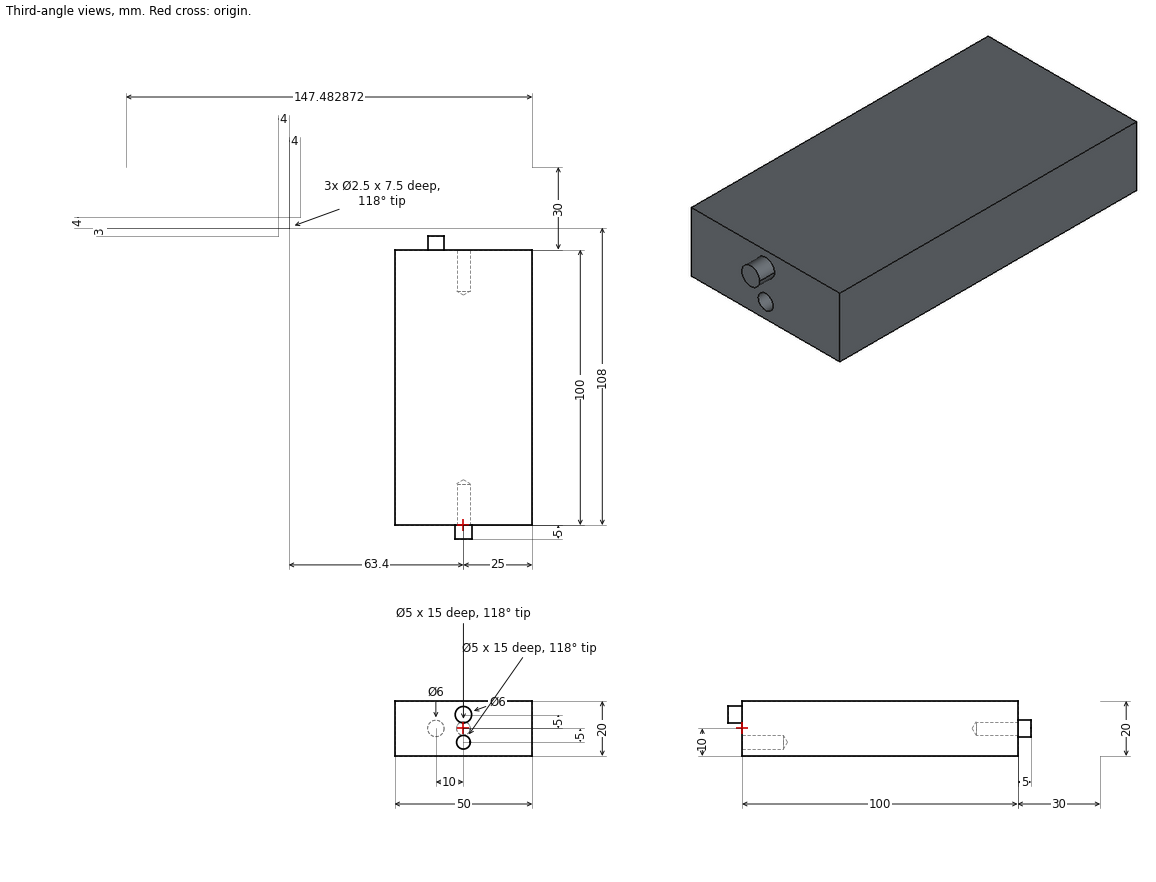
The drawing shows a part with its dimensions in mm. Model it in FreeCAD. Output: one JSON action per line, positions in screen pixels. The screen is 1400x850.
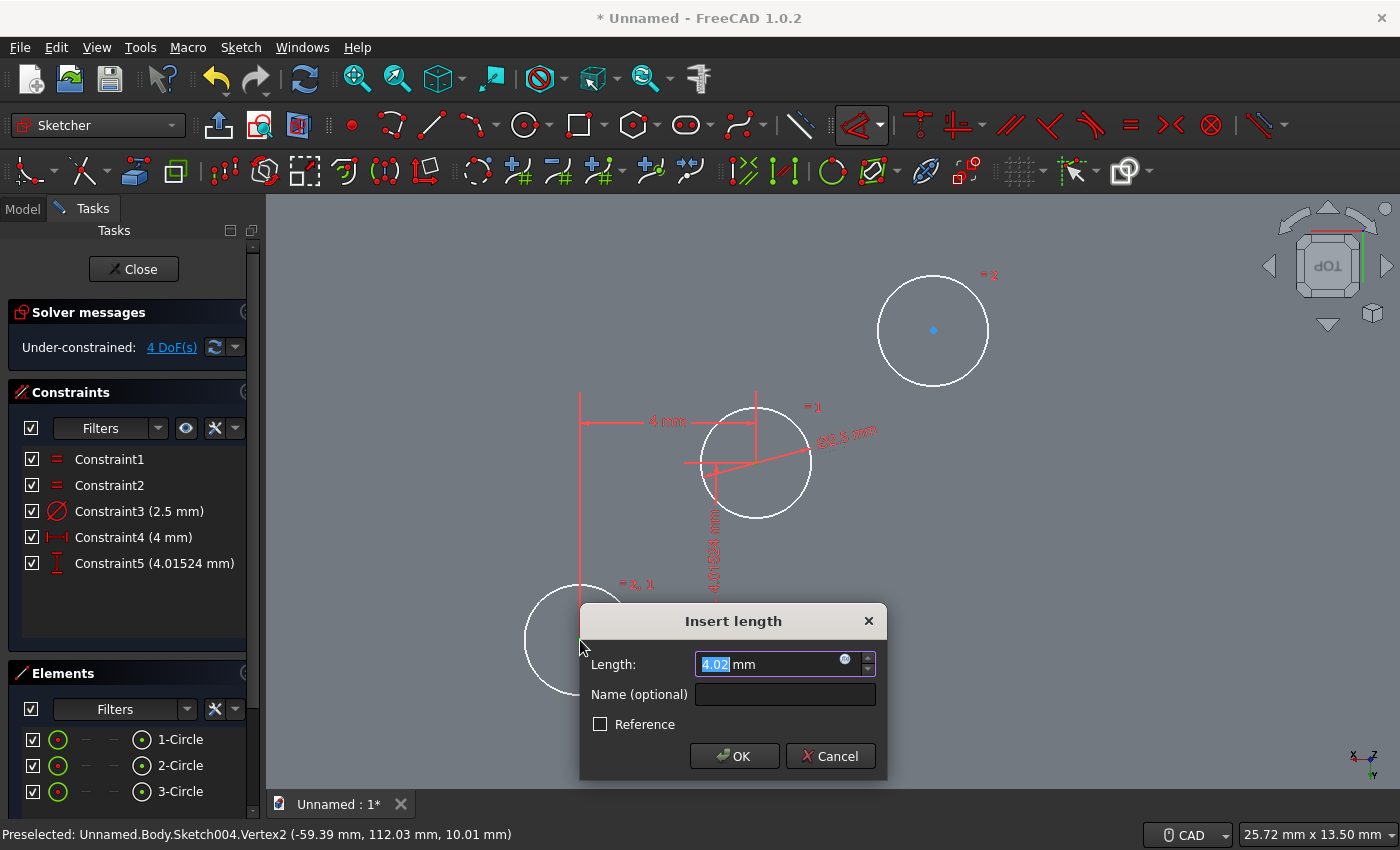
{"action": "type", "text": "4"}
{"action": "key", "text": "Return"}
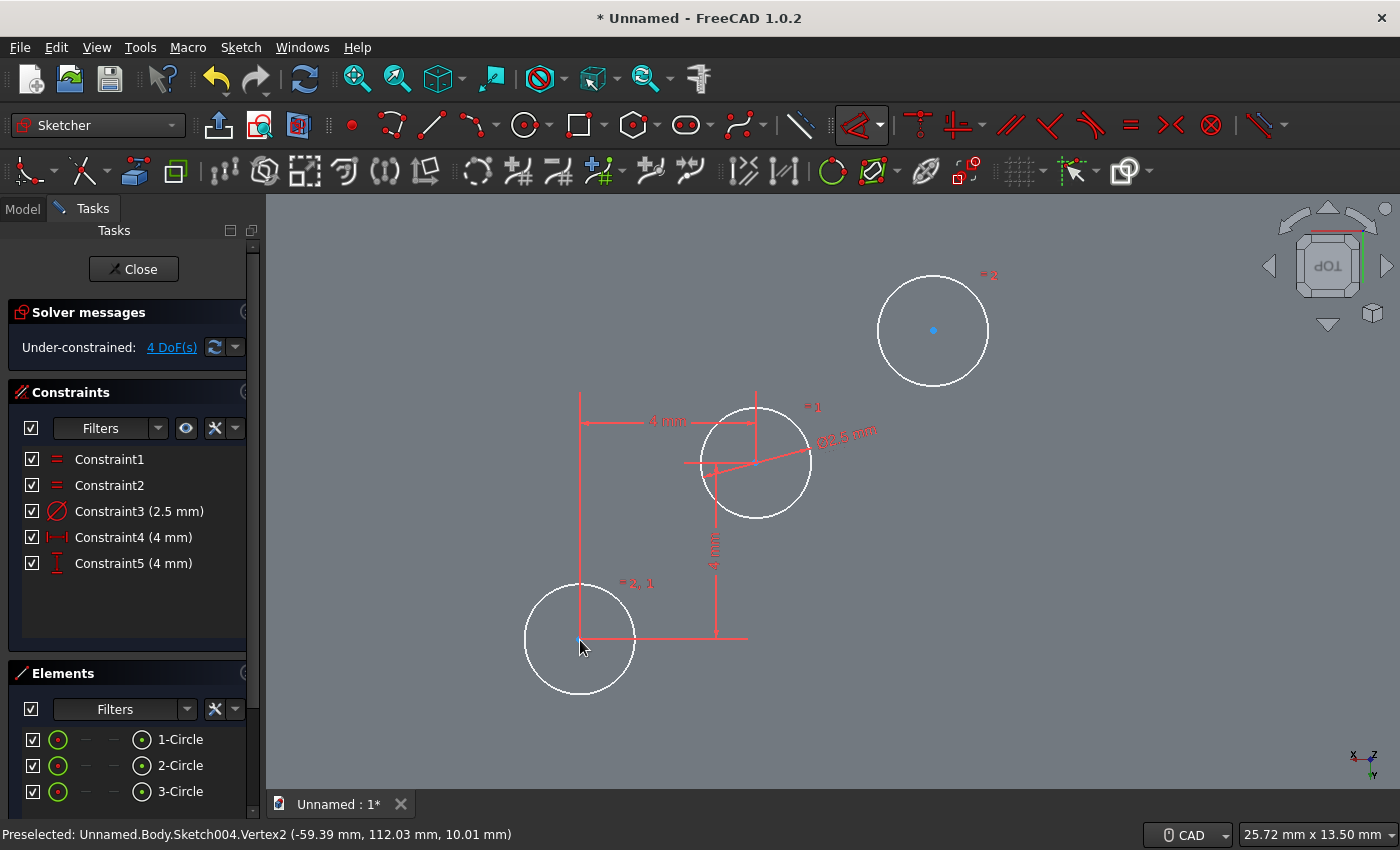
{"action": "left_click", "coordinate": [756, 463]}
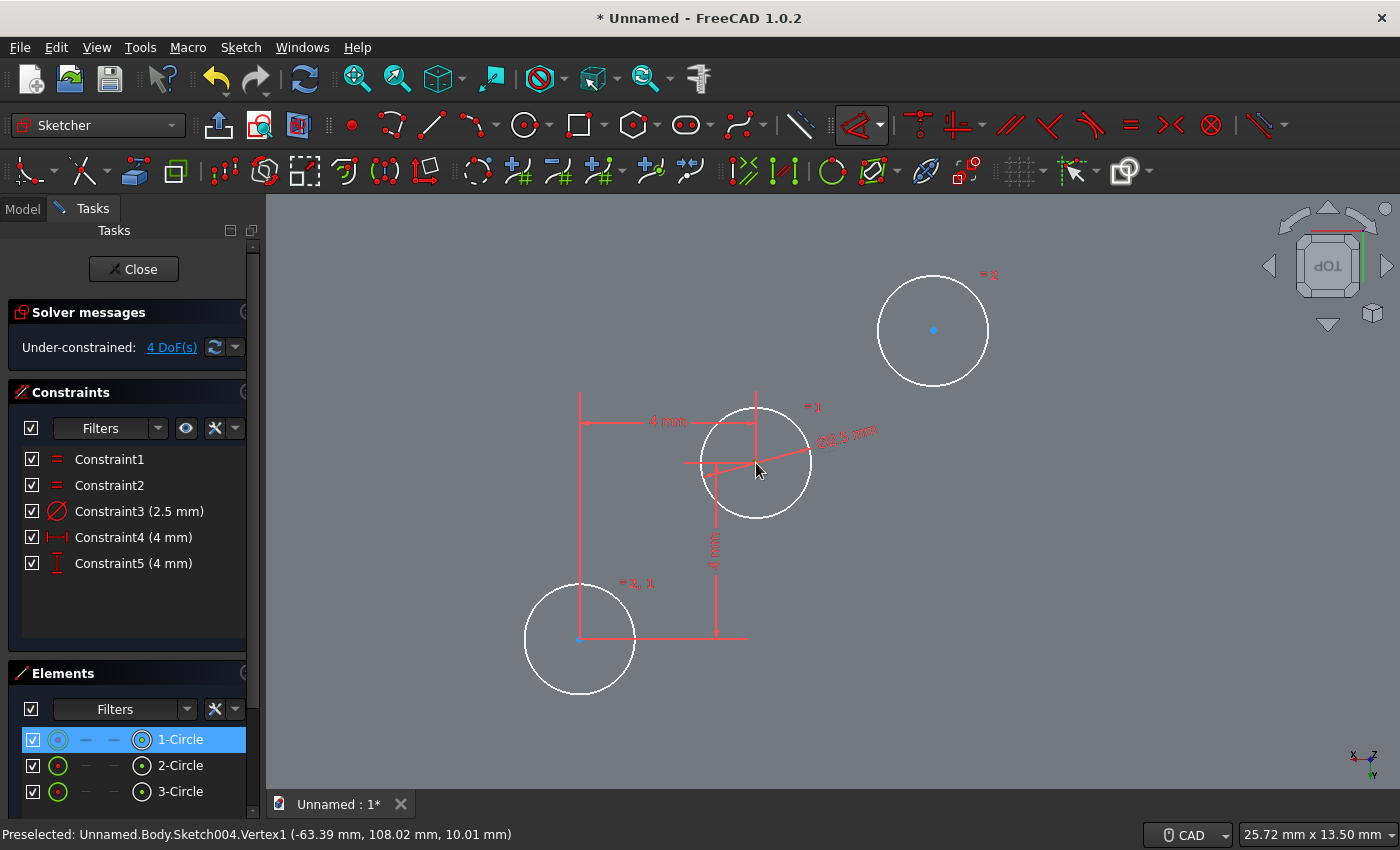
{"action": "left_click", "coordinate": [933, 331]}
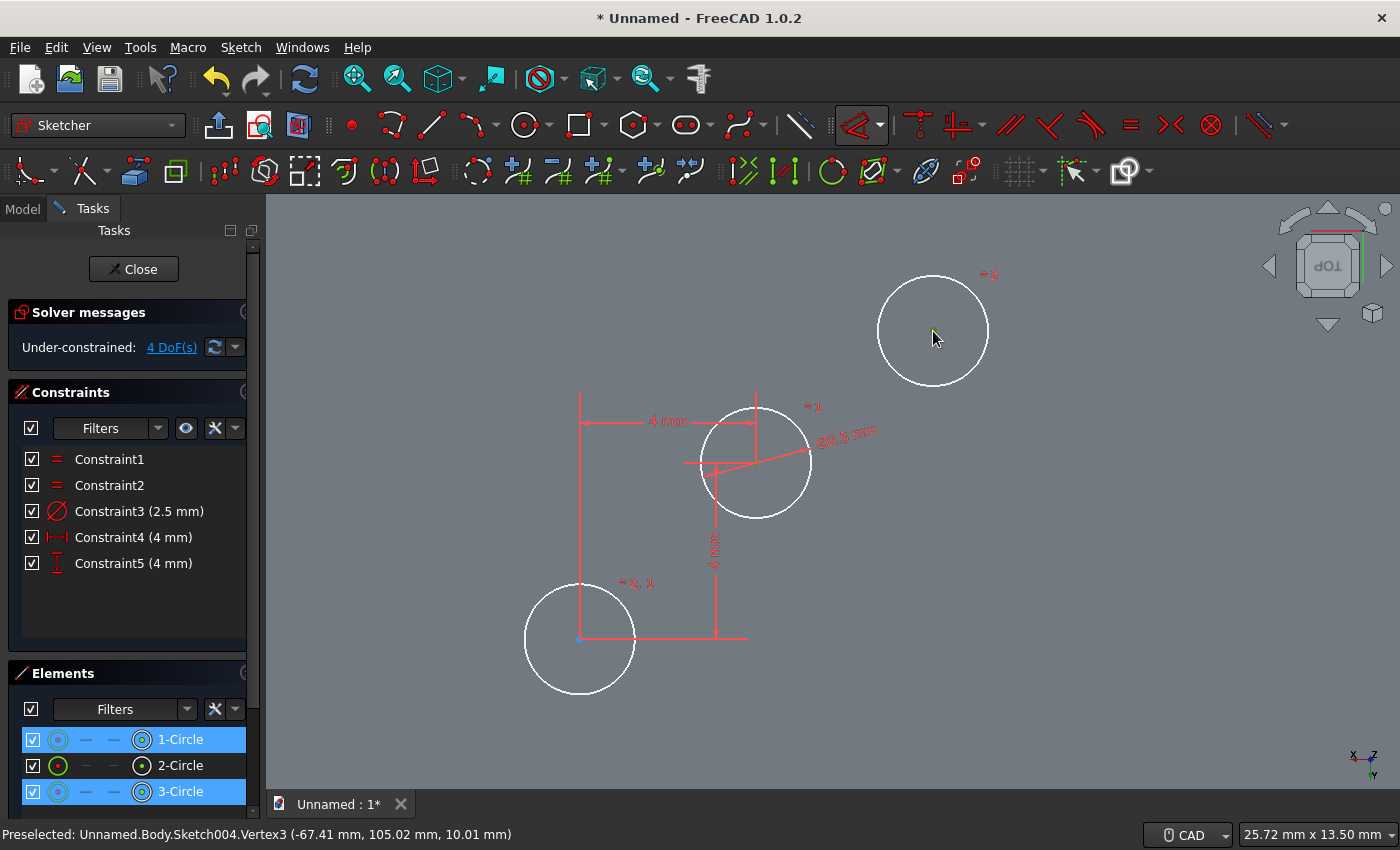
{"action": "key", "text": "l"}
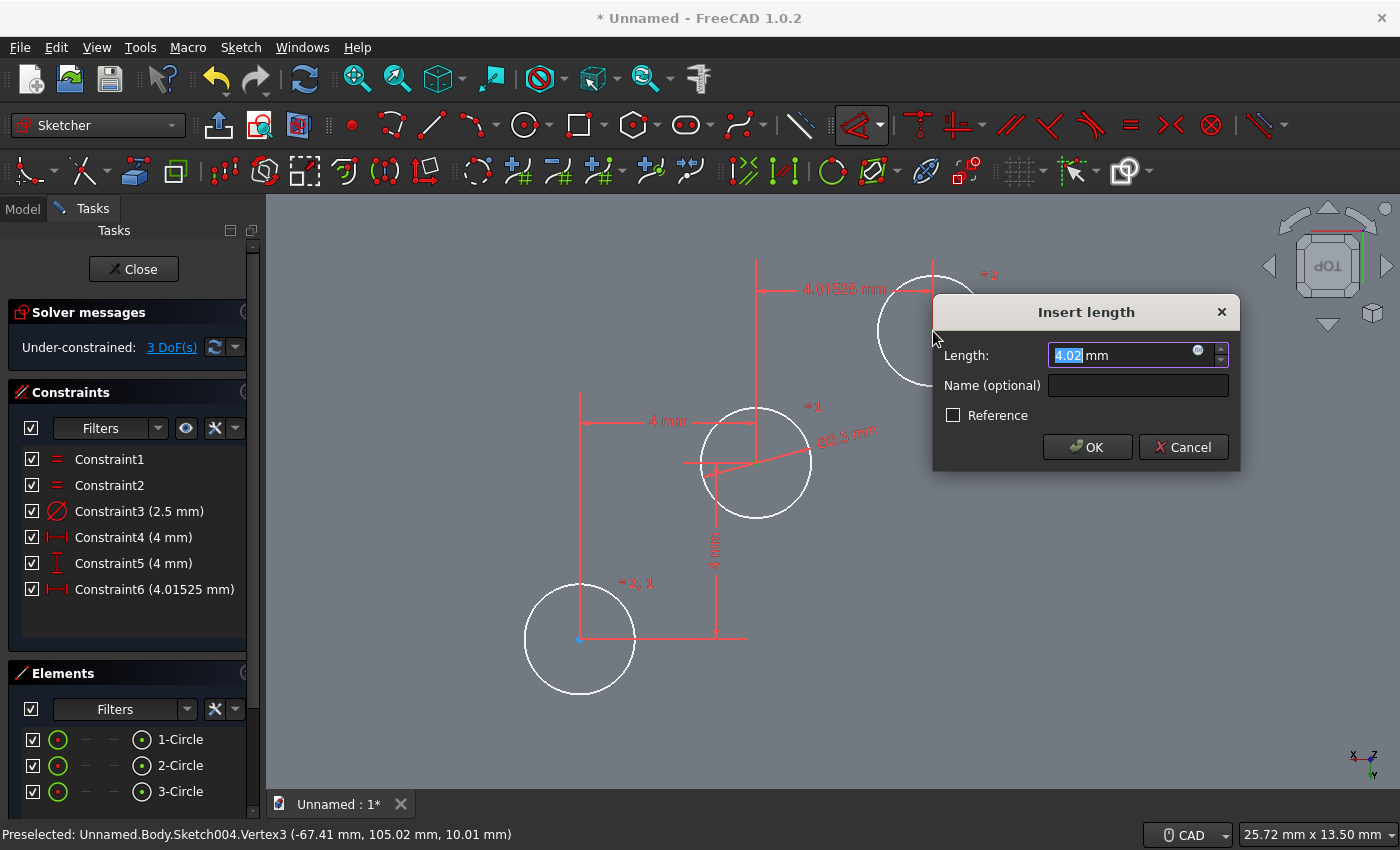
{"action": "type", "text": "4"}
{"action": "key", "text": "Return"}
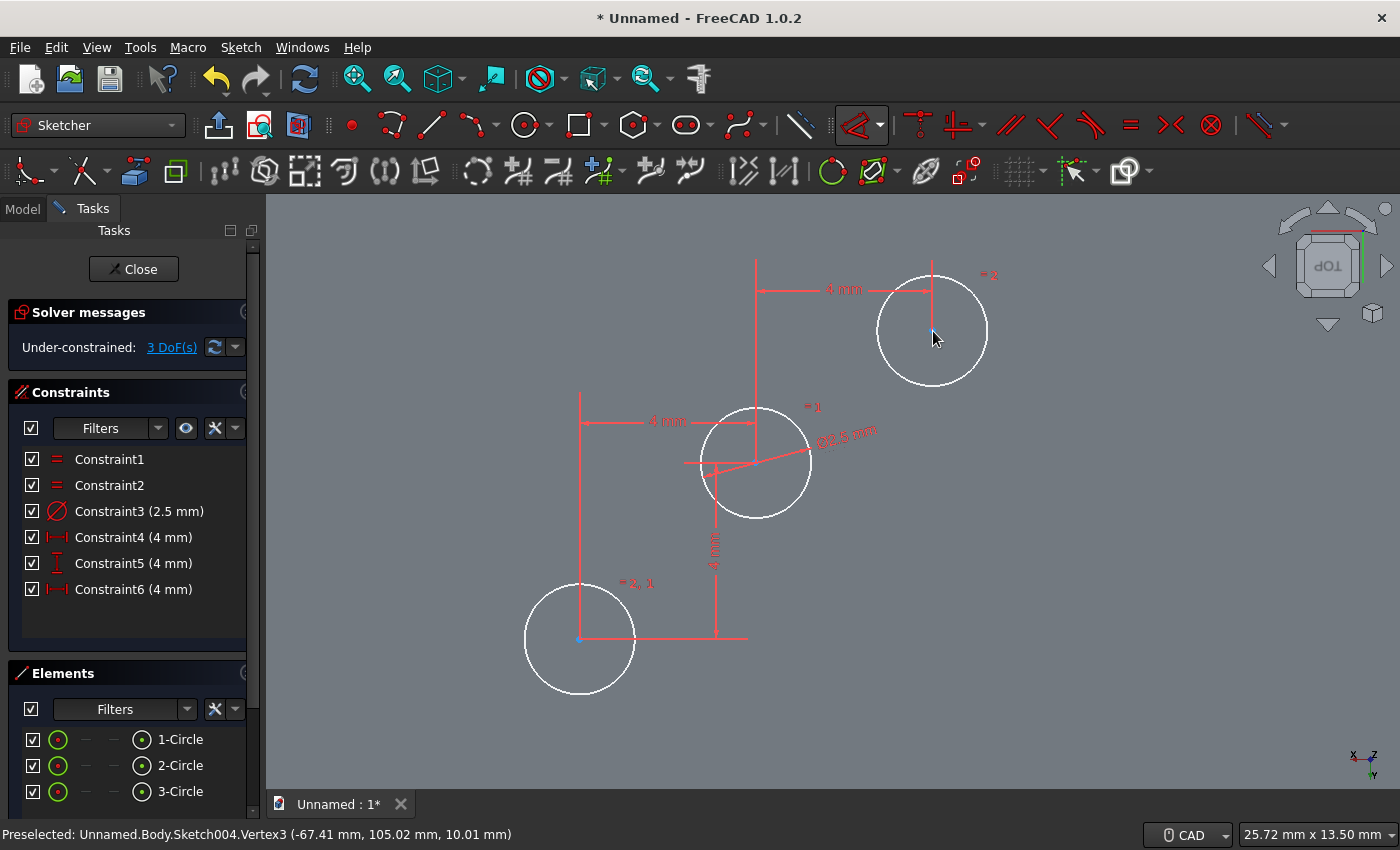
{"action": "left_click", "coordinate": [756, 463]}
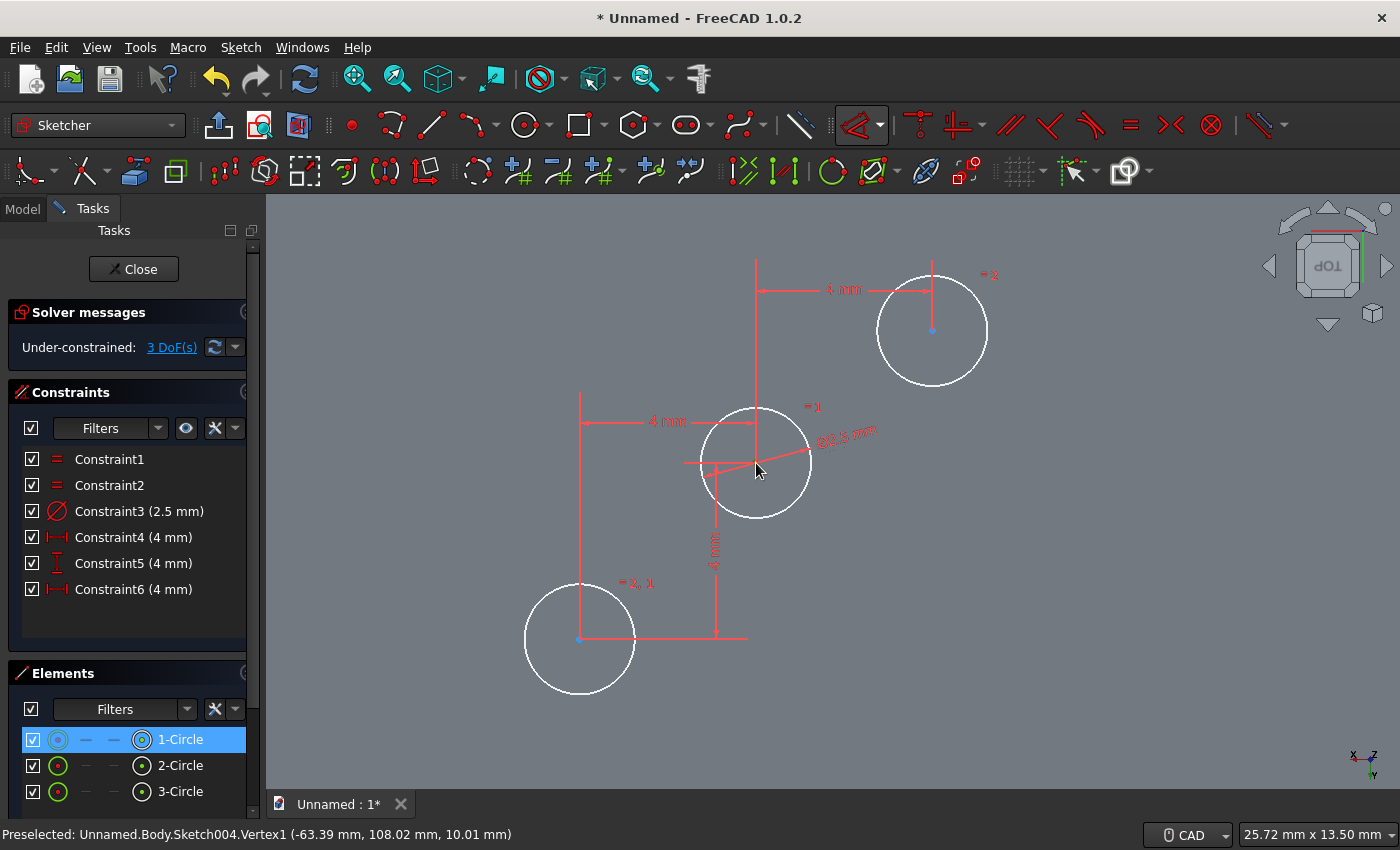
{"action": "left_click", "coordinate": [932, 331]}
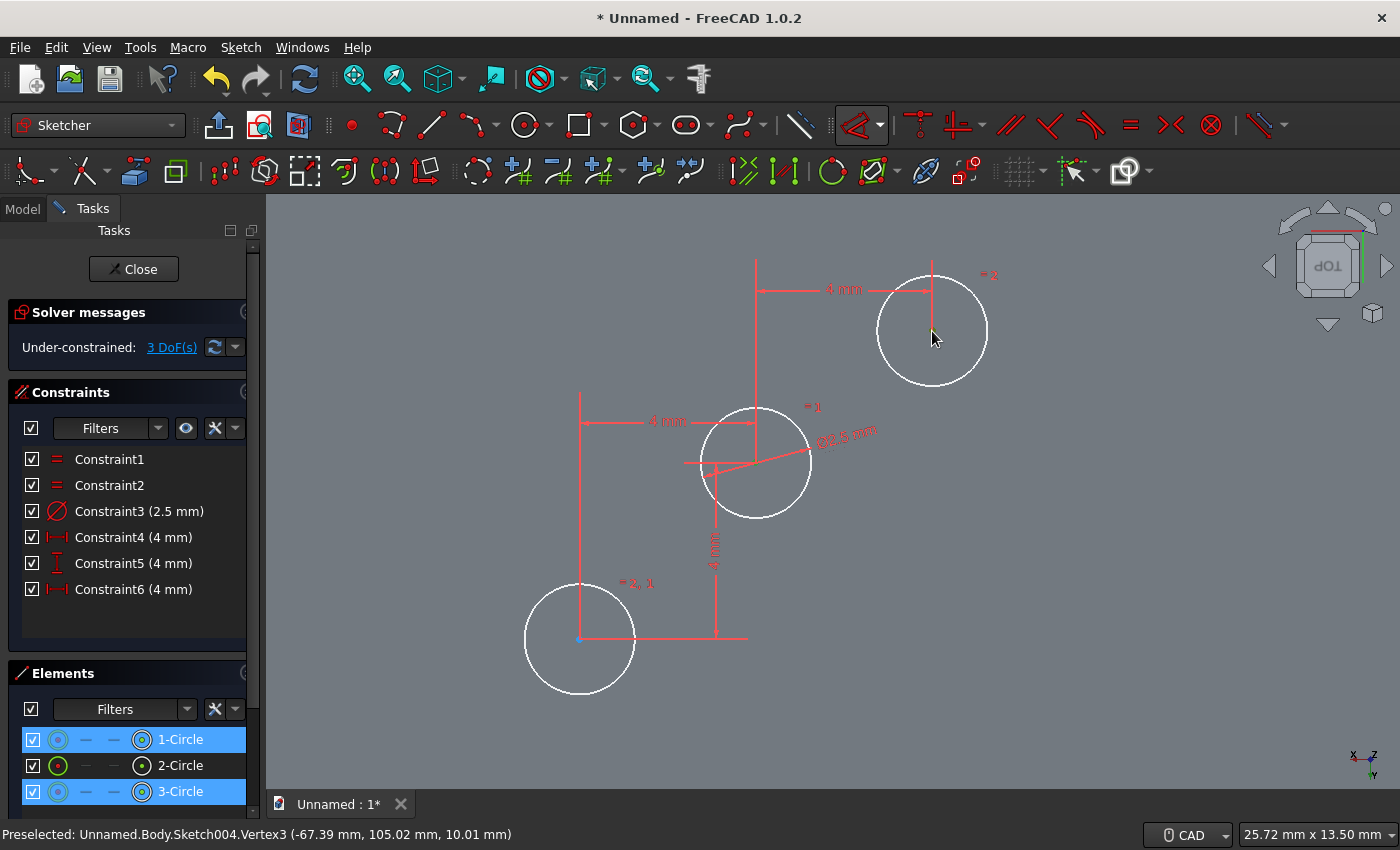
{"action": "key", "text": "i"}